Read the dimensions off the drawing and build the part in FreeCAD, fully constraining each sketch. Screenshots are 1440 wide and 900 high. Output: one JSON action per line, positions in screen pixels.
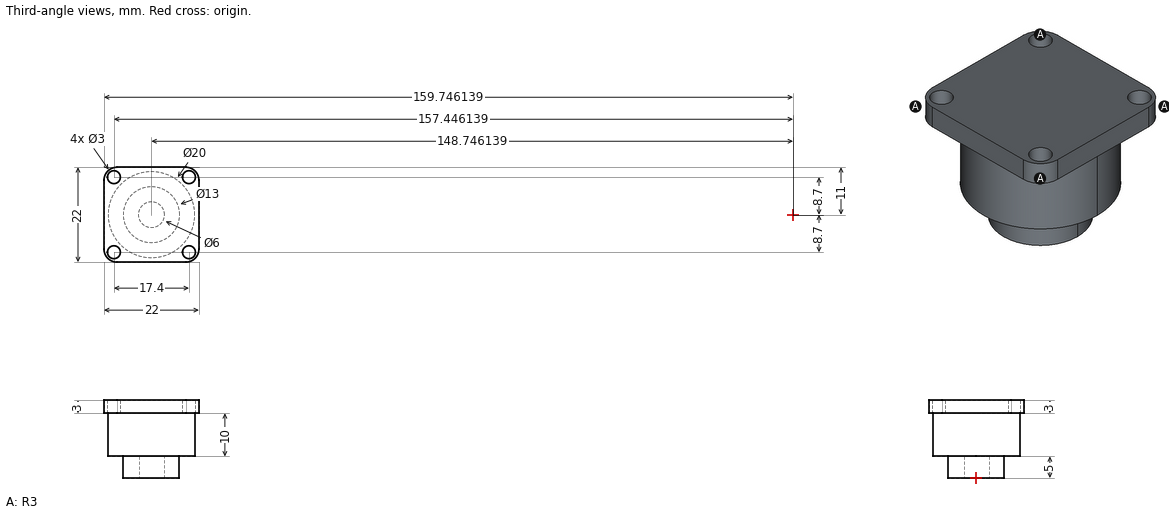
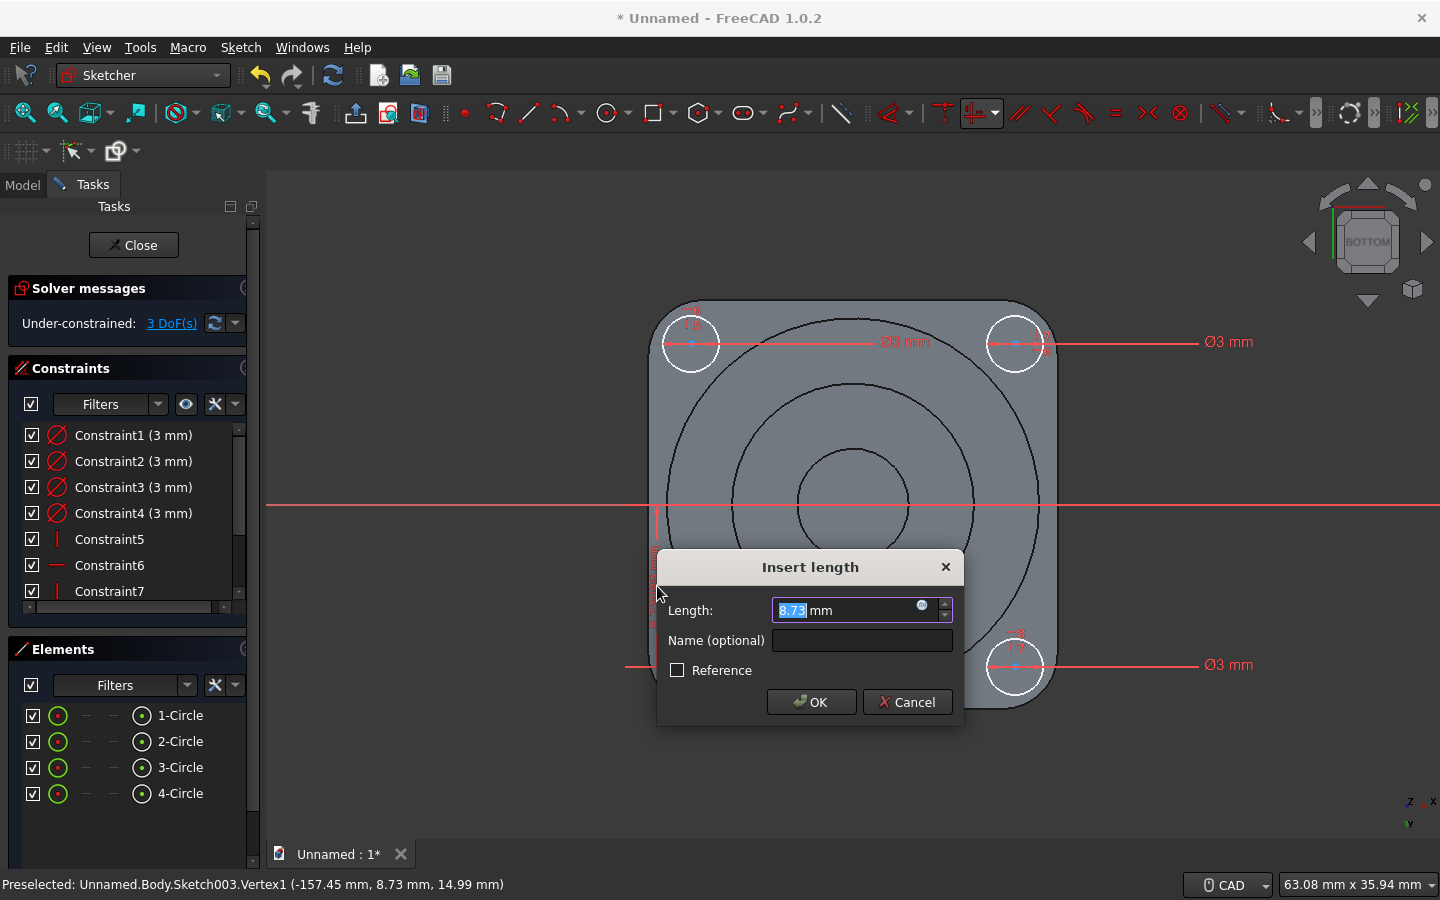
{"action": "type", "text": "8.7"}
{"action": "key", "text": "Return"}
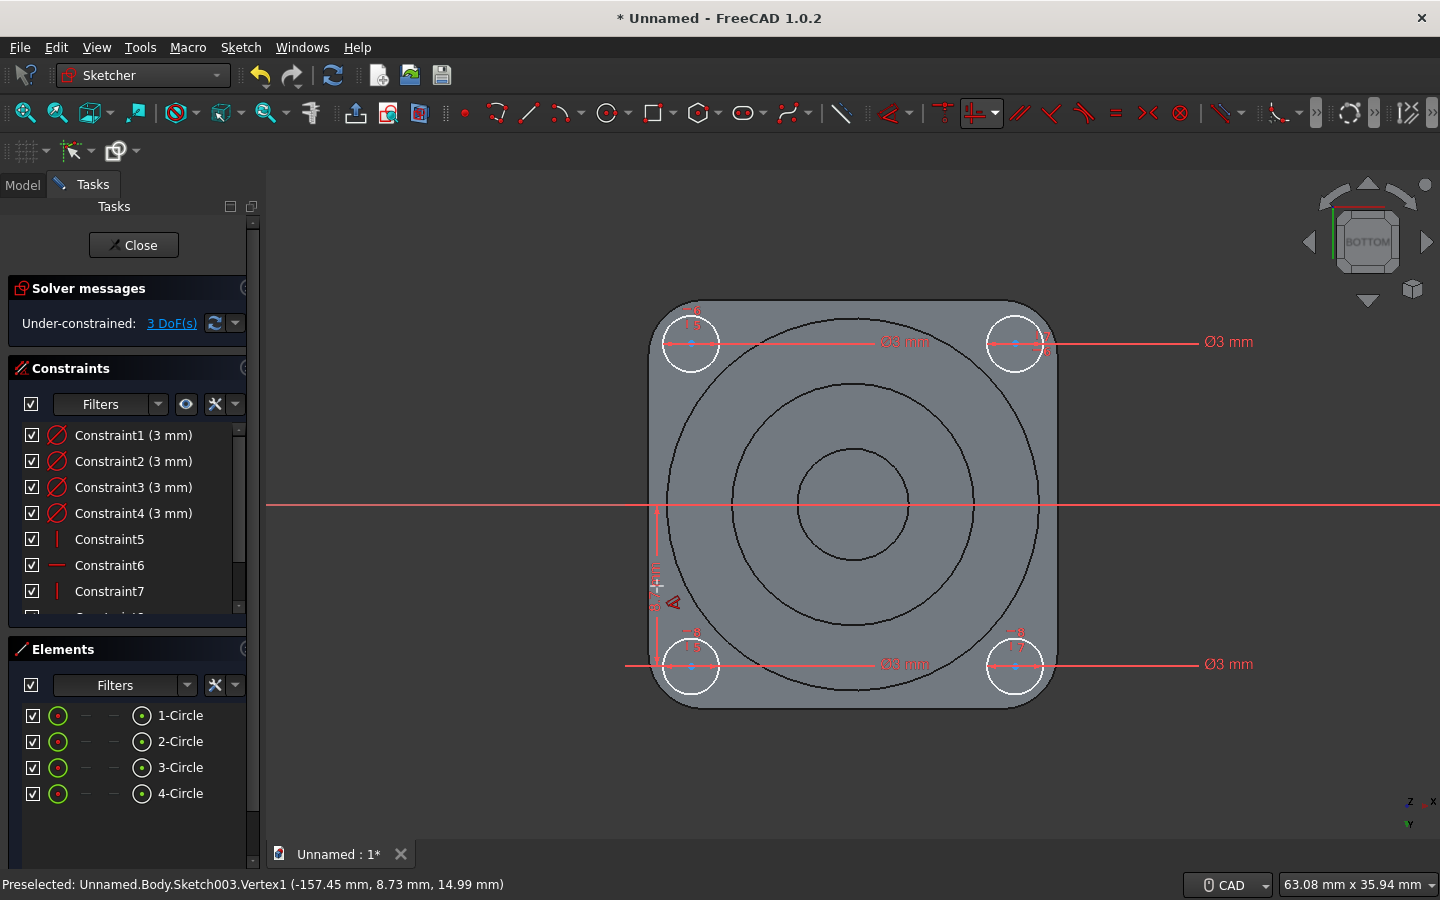
{"action": "left_click", "coordinate": [691, 344]}
{"action": "left_click", "coordinate": [657, 424]}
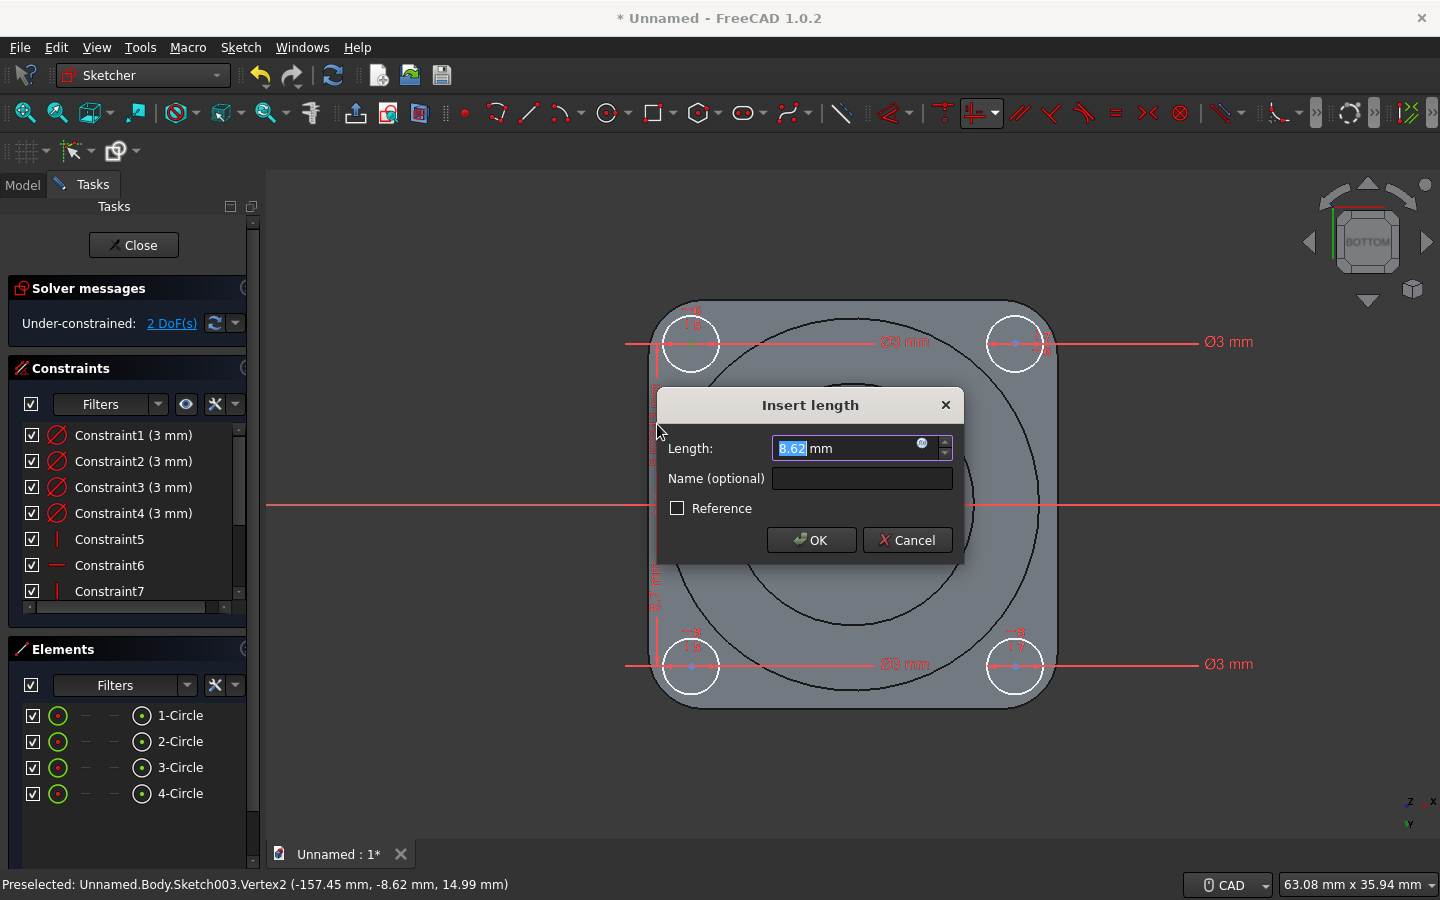
{"action": "type", "text": "8.7"}
{"action": "key", "text": "Return"}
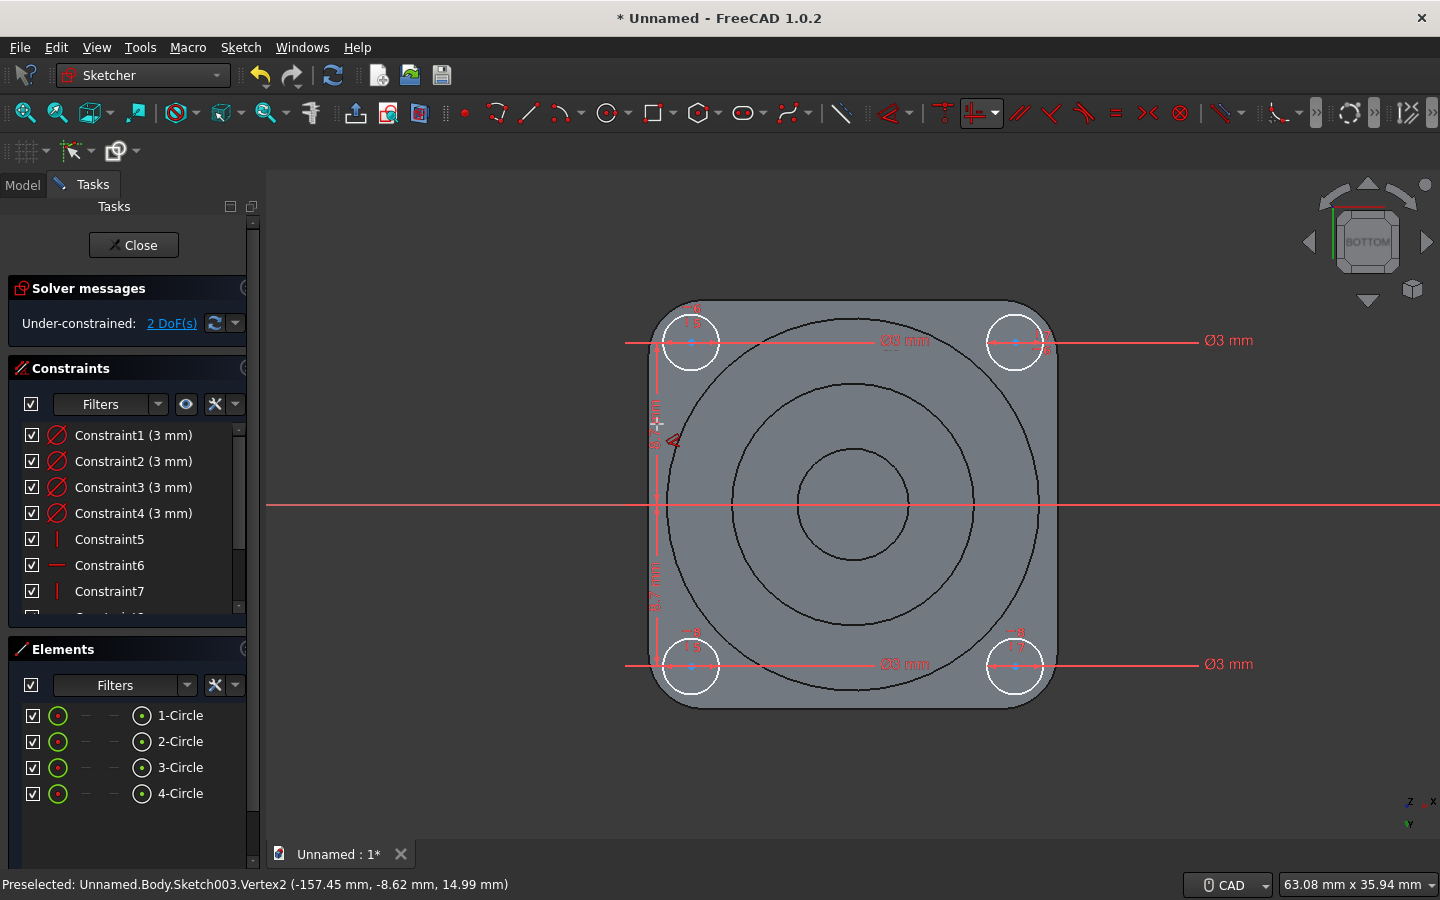
{"action": "left_click", "coordinate": [691, 343]}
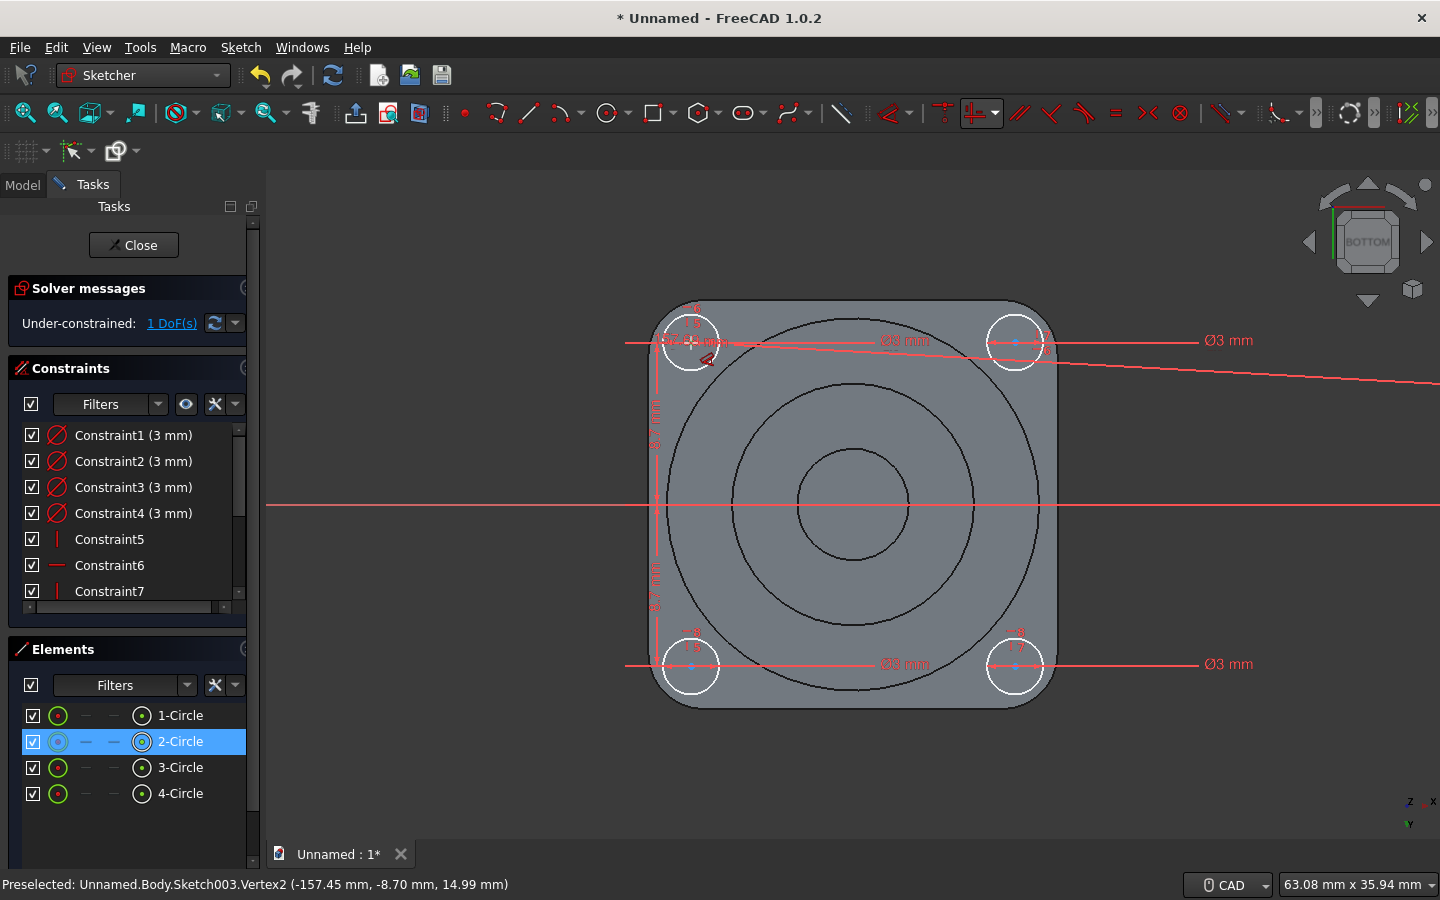
{"action": "left_click", "coordinate": [1015, 343]}
{"action": "left_click", "coordinate": [853, 309]}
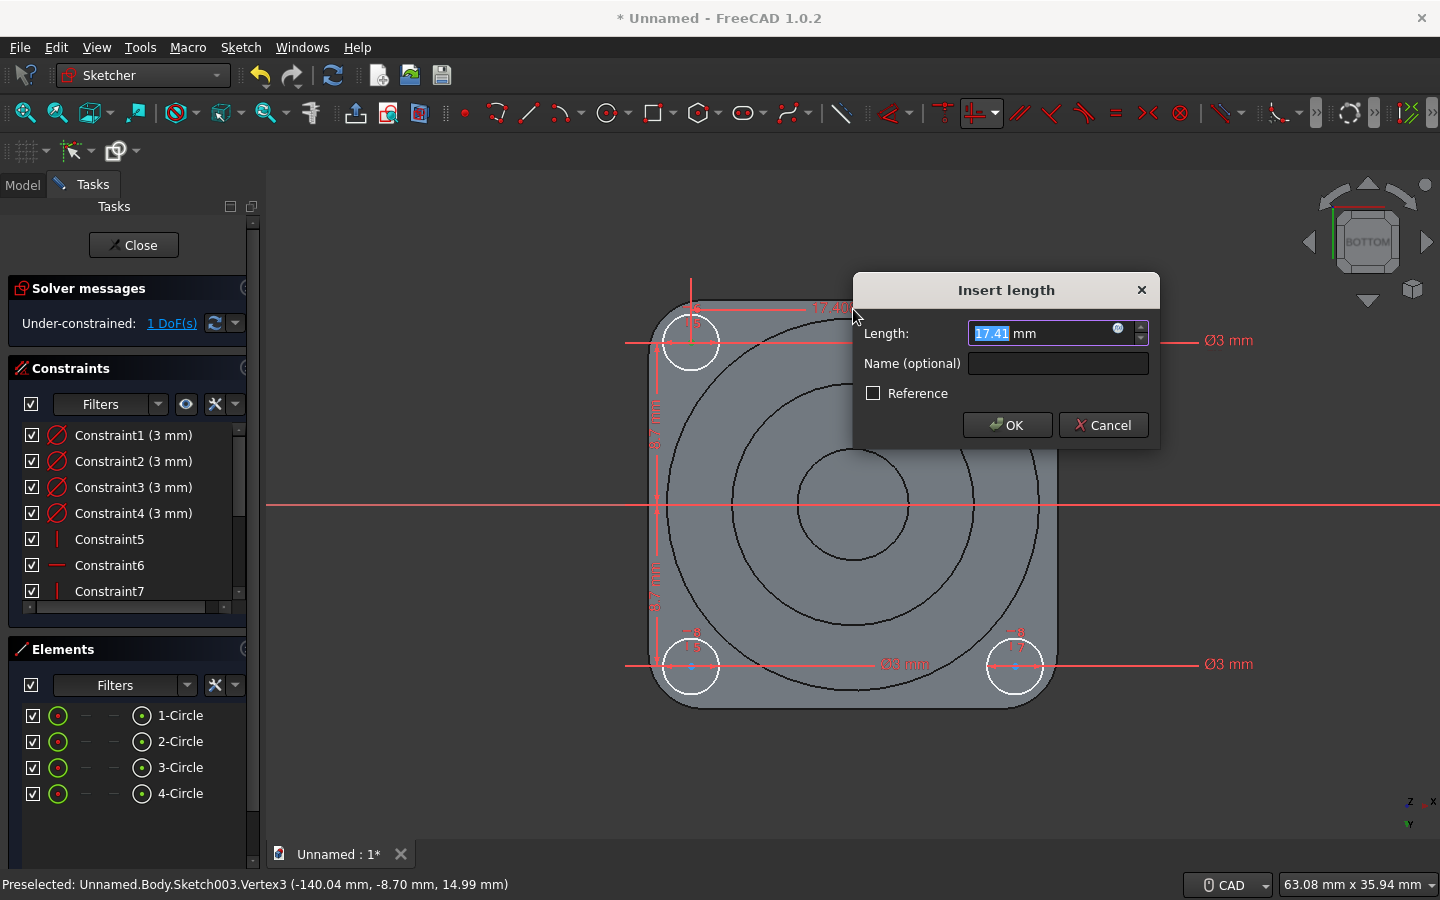
{"action": "type", "text": "17.4"}
{"action": "key", "text": "Return"}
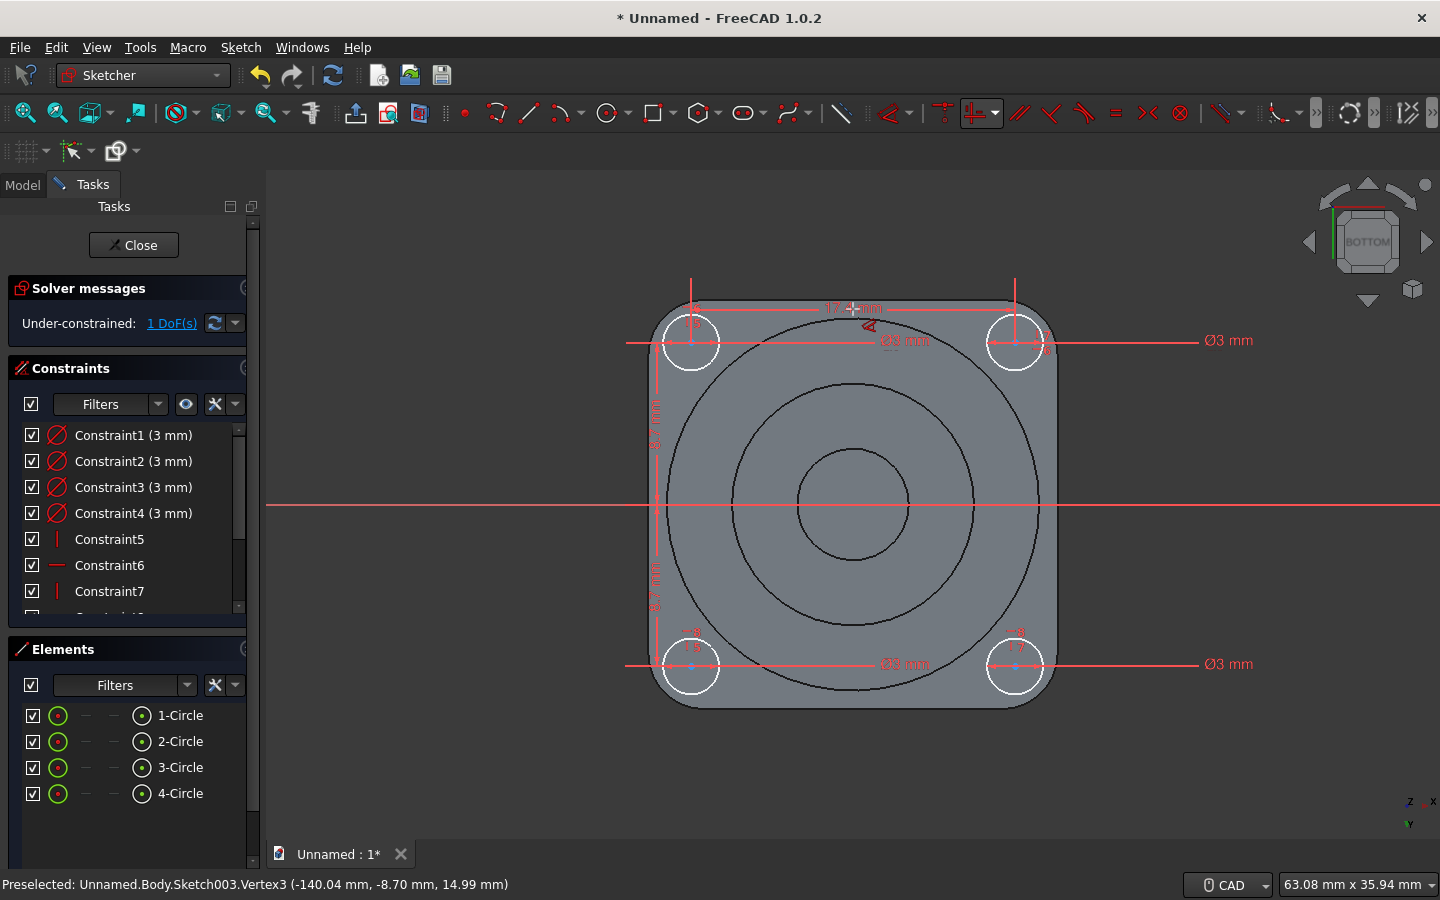
{"action": "left_click", "coordinate": [691, 666]}
{"action": "left_click", "coordinate": [983, 700]}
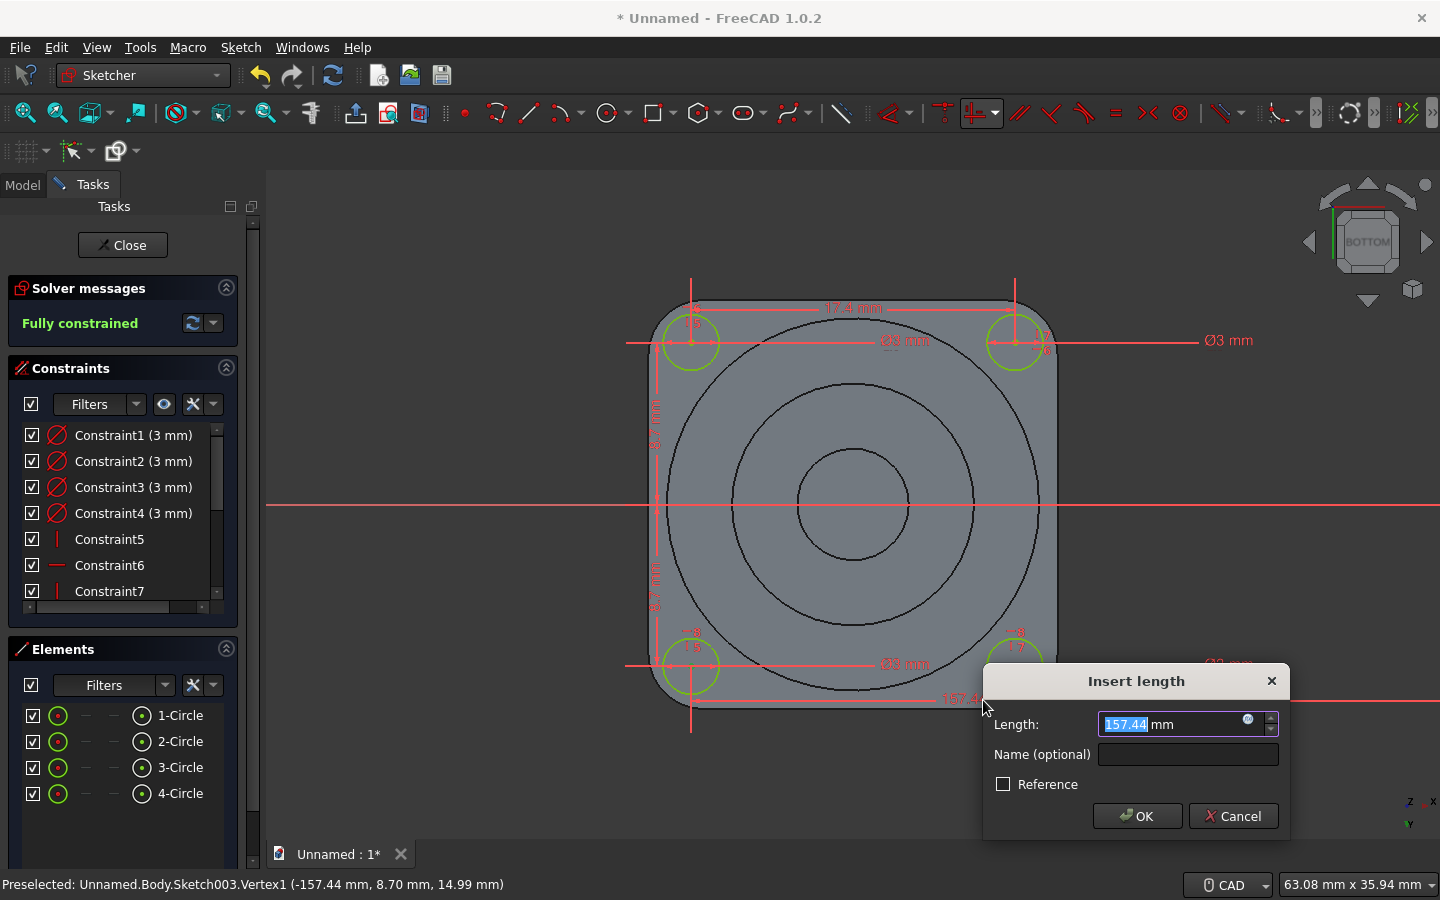
{"action": "type", "text": "157.446139"}
{"action": "key", "text": "Return"}
{"action": "key", "text": "Escape"}